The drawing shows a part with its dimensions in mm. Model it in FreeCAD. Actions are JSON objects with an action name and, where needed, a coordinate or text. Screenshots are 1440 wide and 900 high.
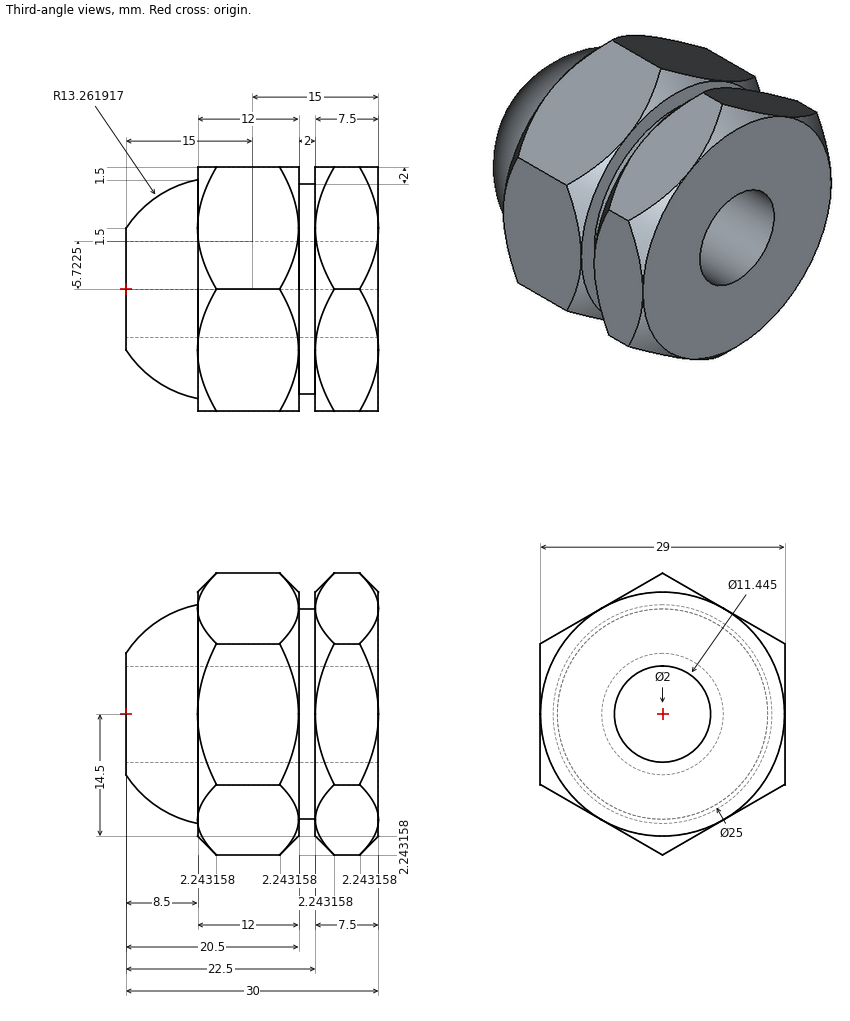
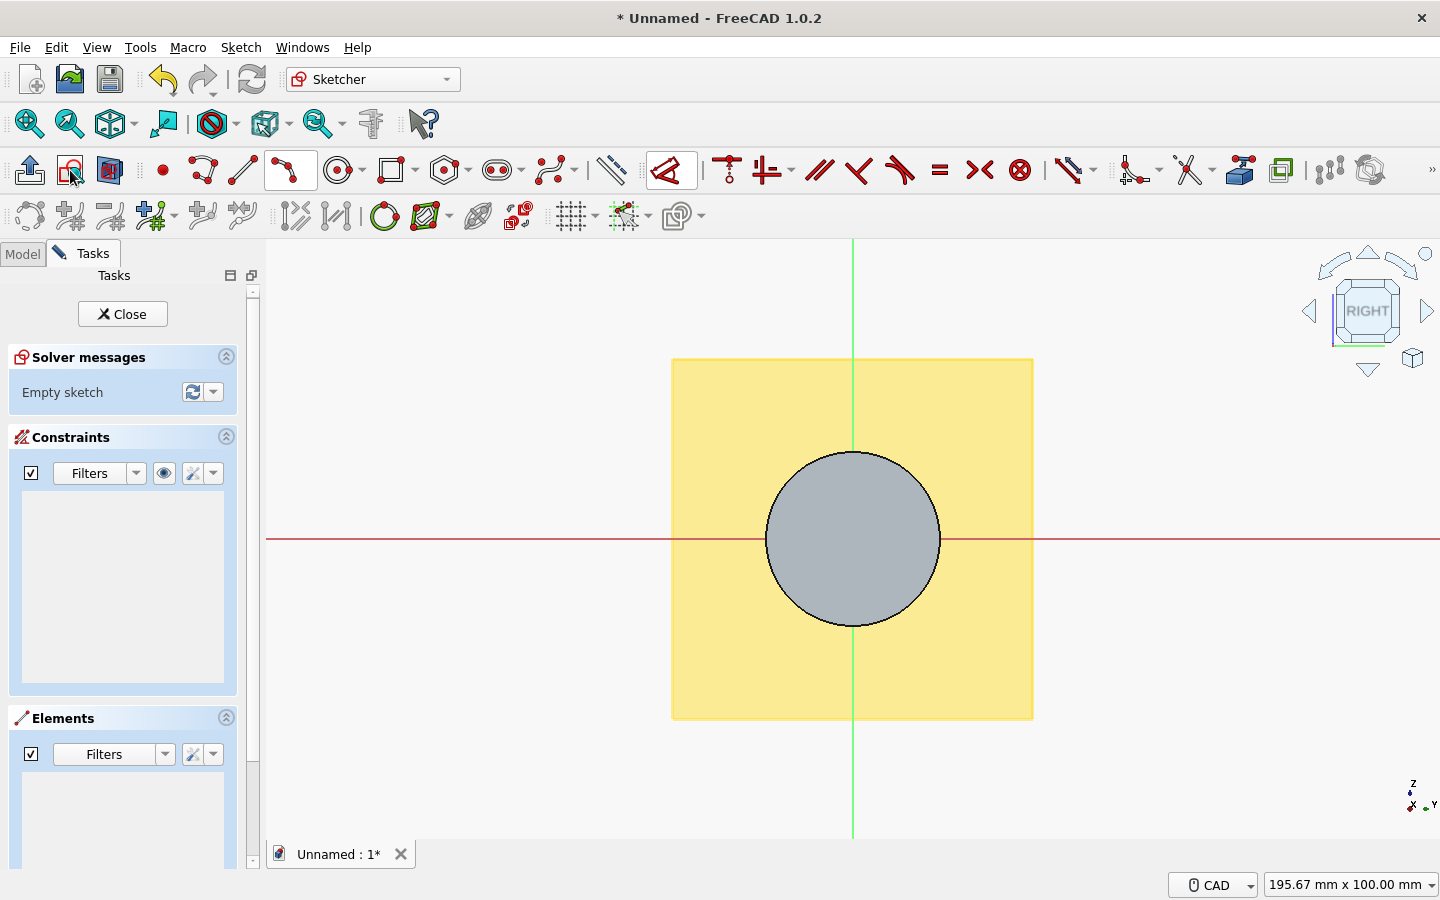
{"action": "left_click", "coordinate": [110, 170]}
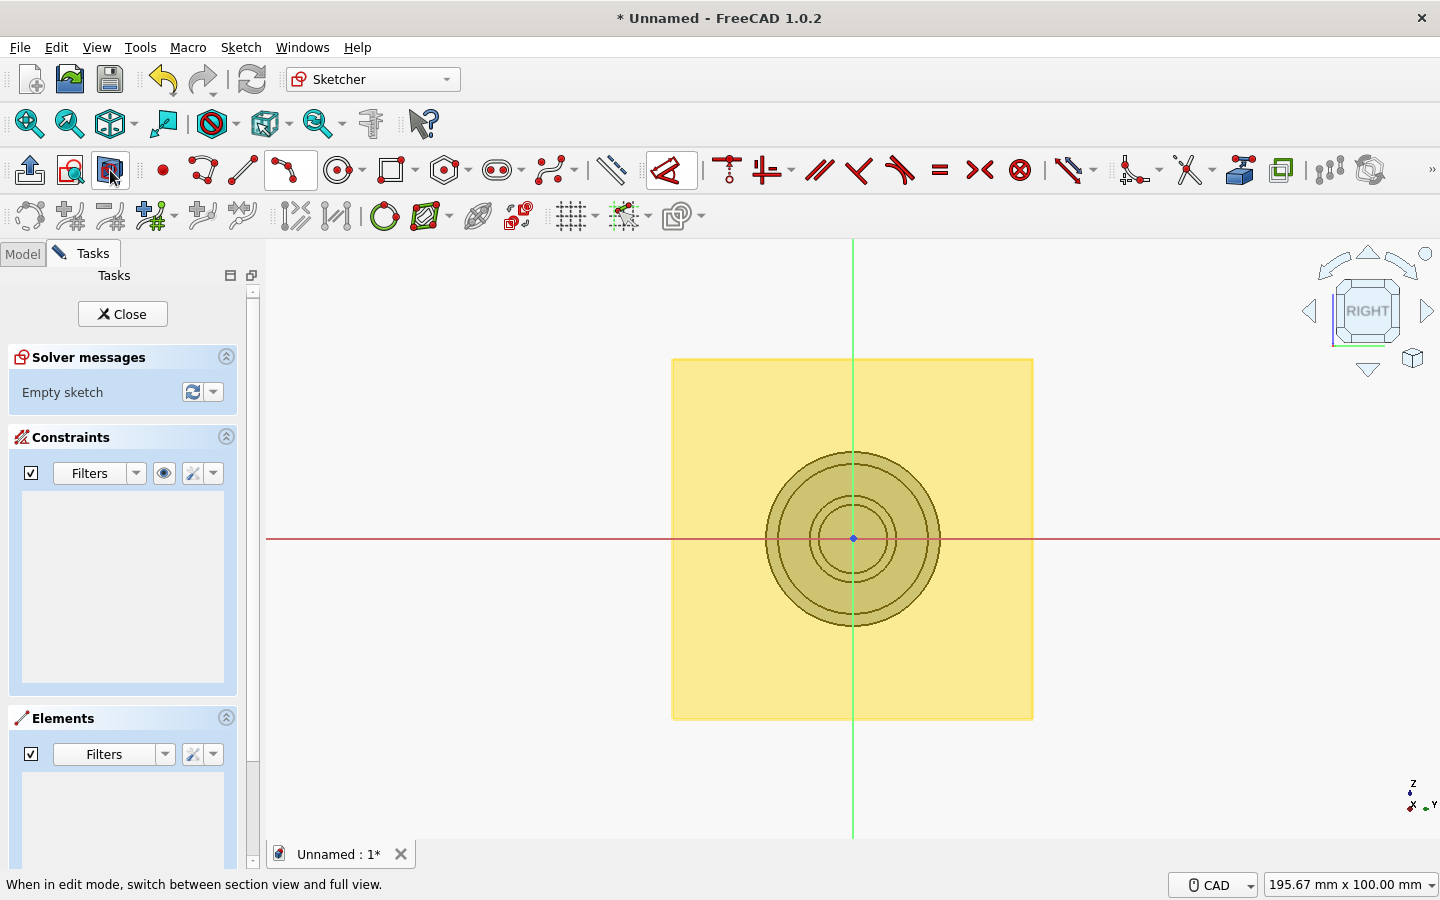
{"action": "scroll", "coordinate": [936, 539], "scroll_direction": "up", "scroll_amount": 3}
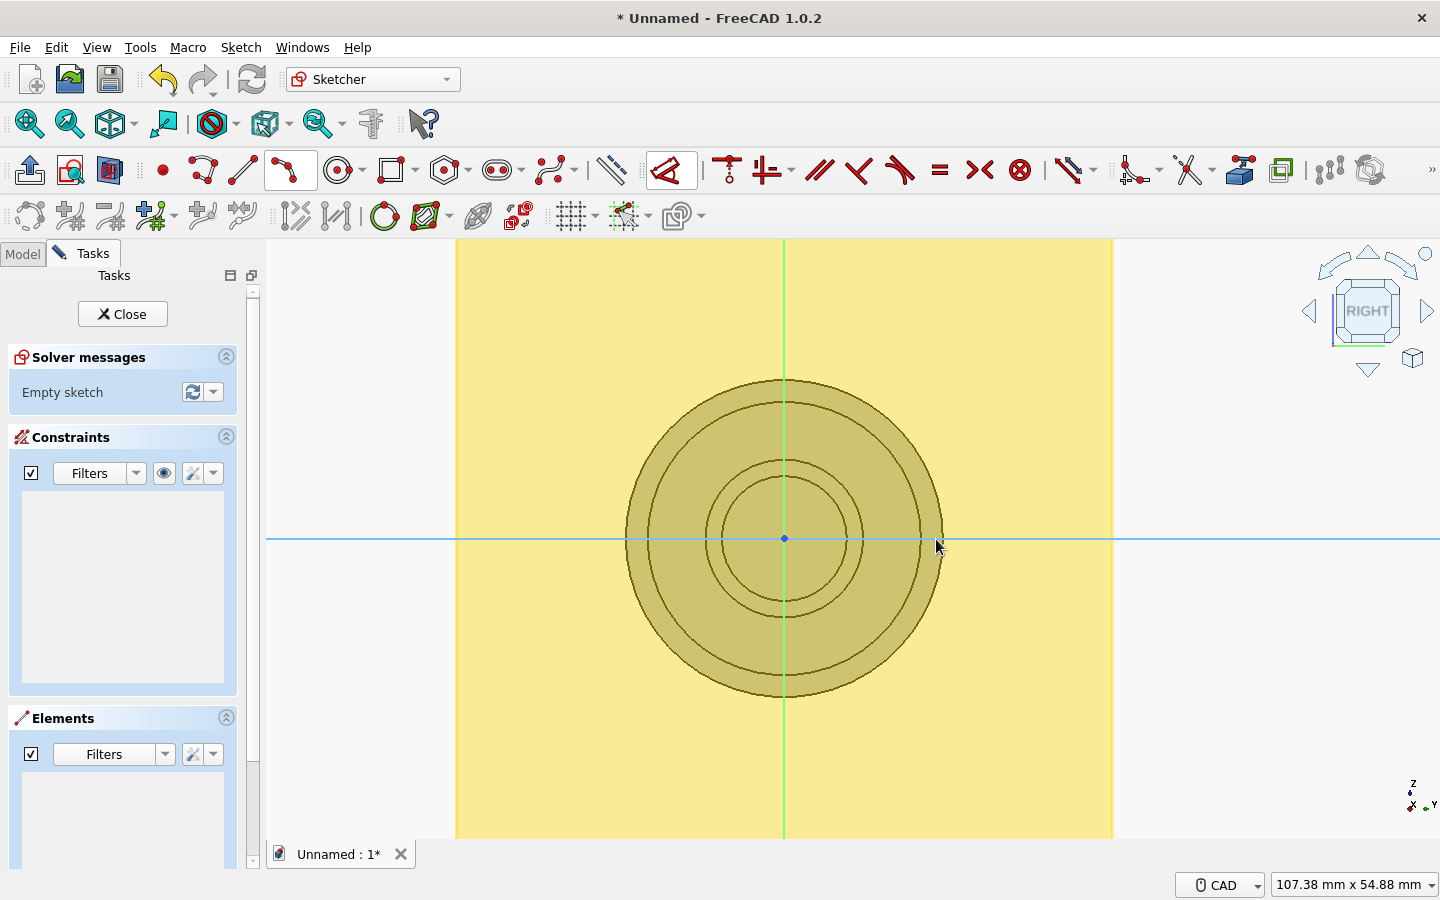
{"action": "left_click", "coordinate": [444, 170]}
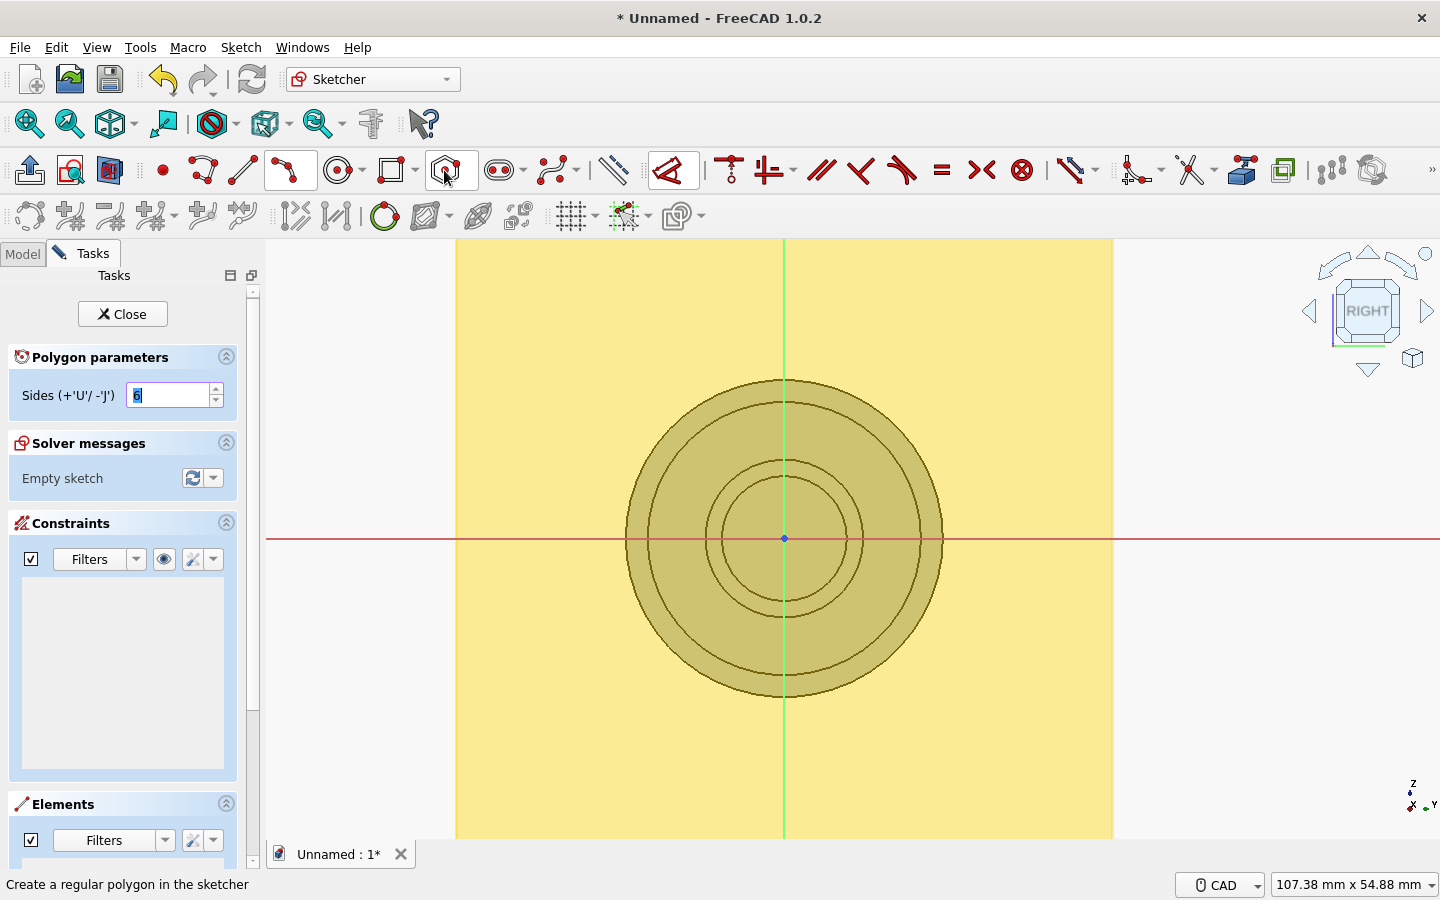
{"action": "left_click", "coordinate": [784, 539]}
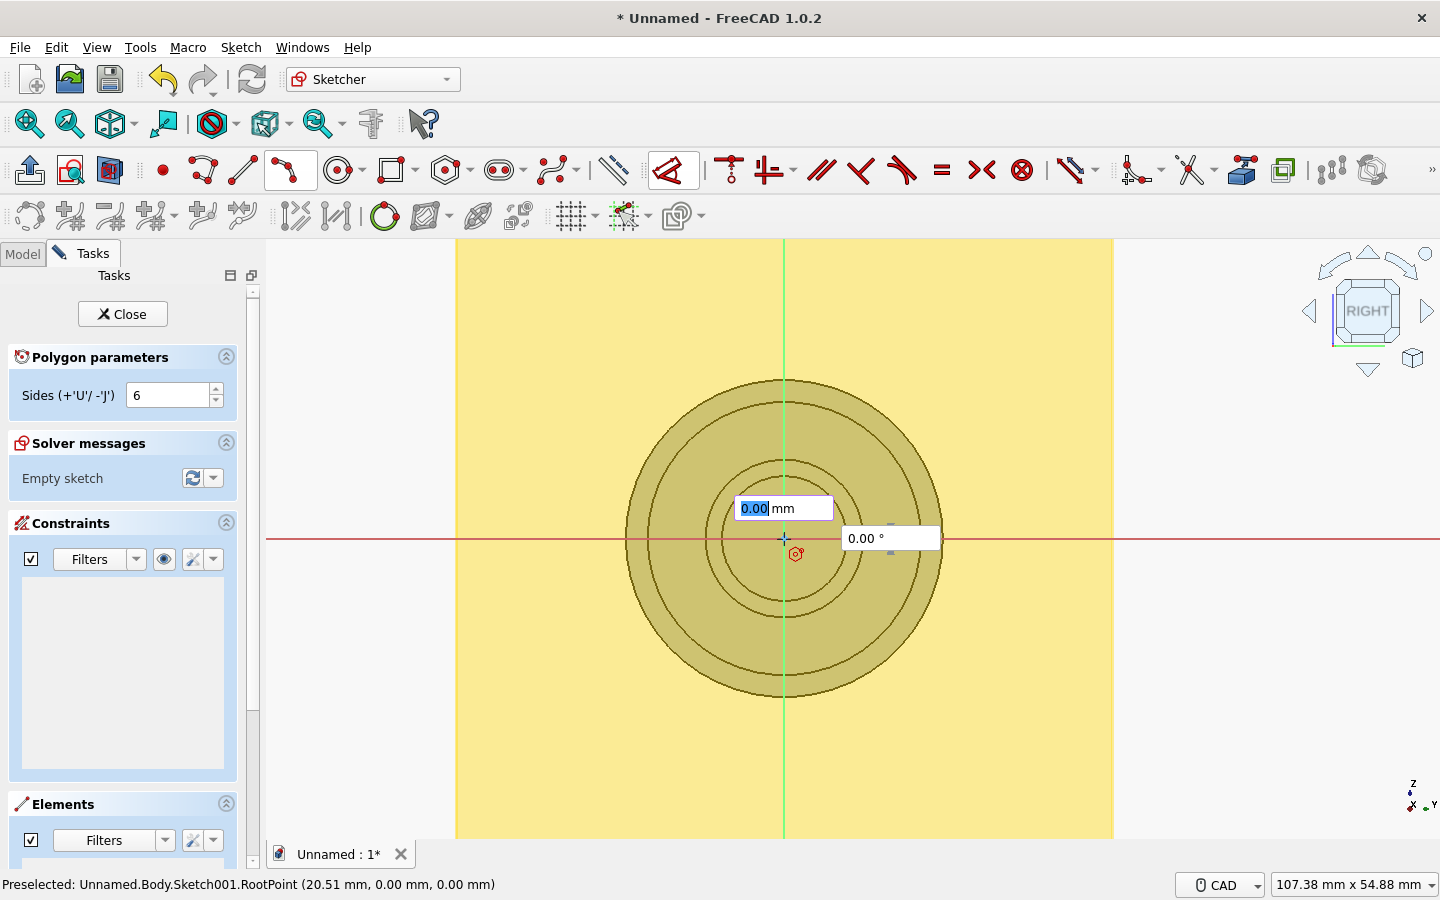
{"action": "left_click", "coordinate": [784, 722]}
{"action": "key", "text": "Escape"}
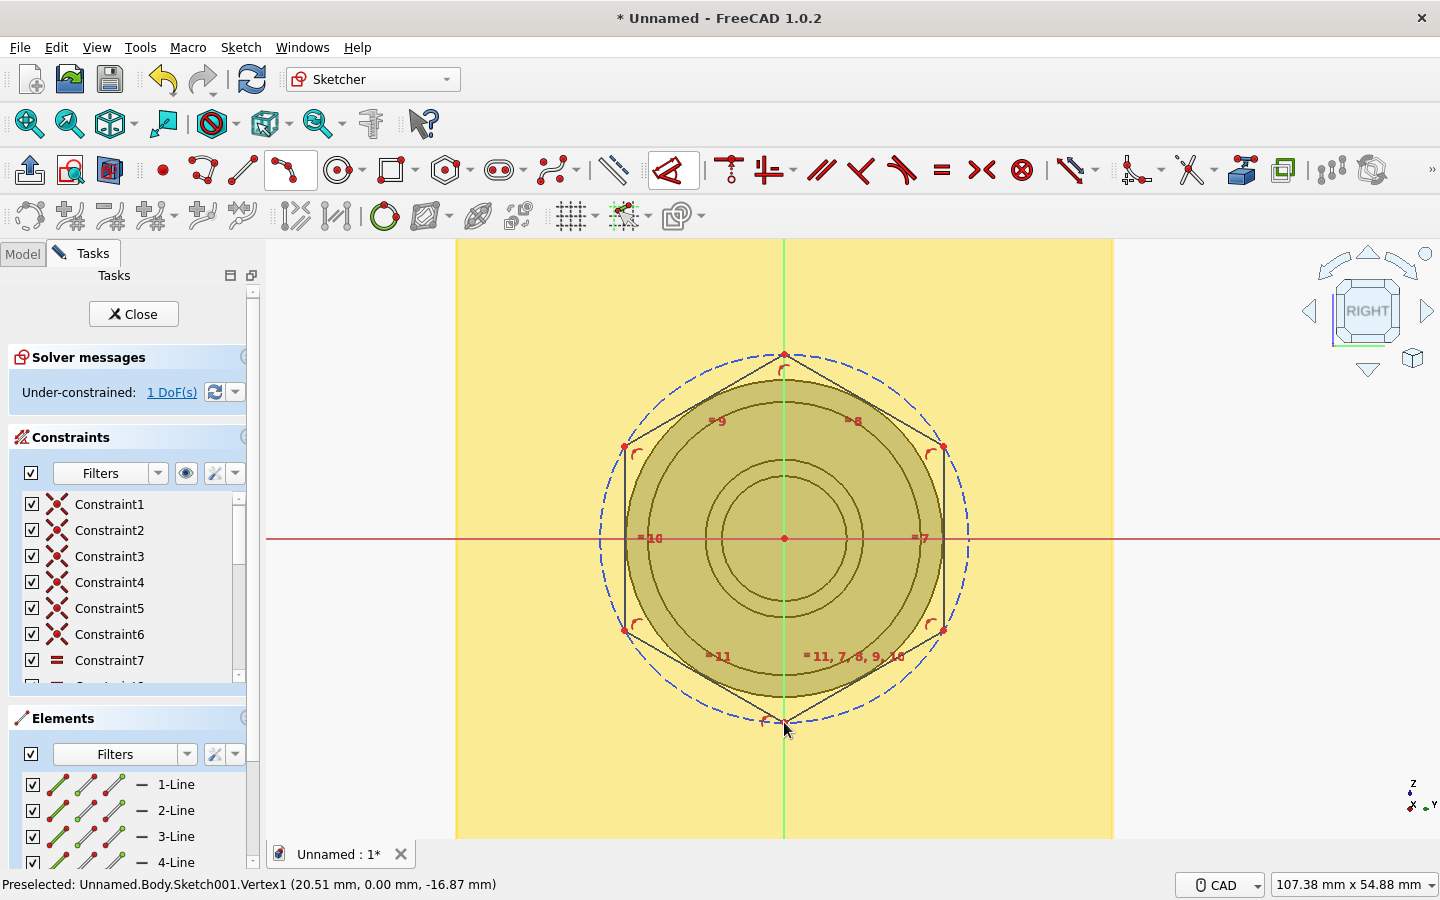
{"action": "key", "text": "g c"}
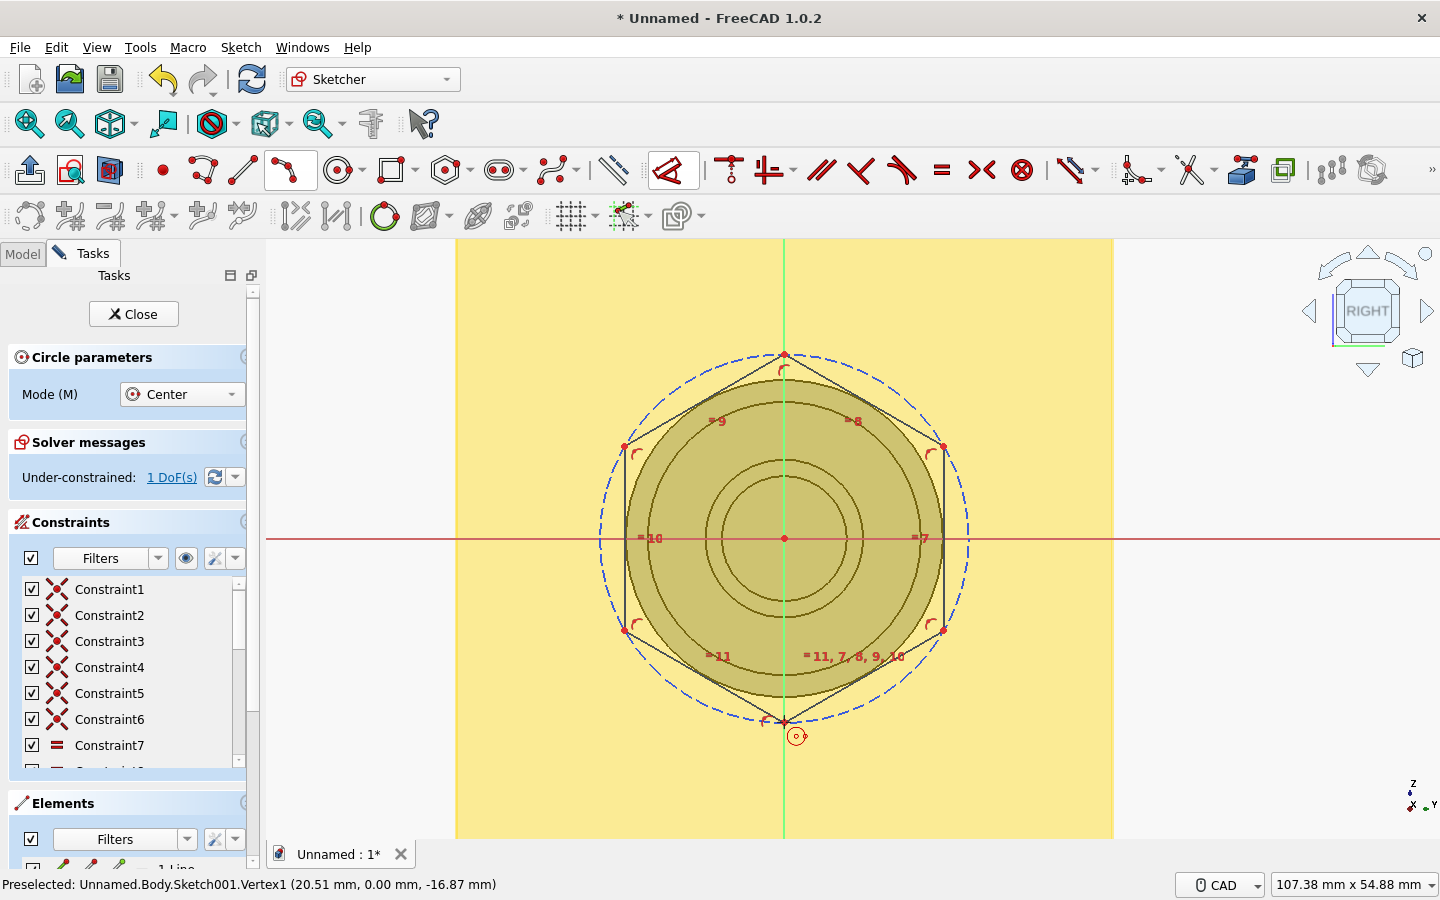
{"action": "left_click", "coordinate": [784, 539]}
{"action": "left_click", "coordinate": [881, 442]}
{"action": "key", "text": "Escape"}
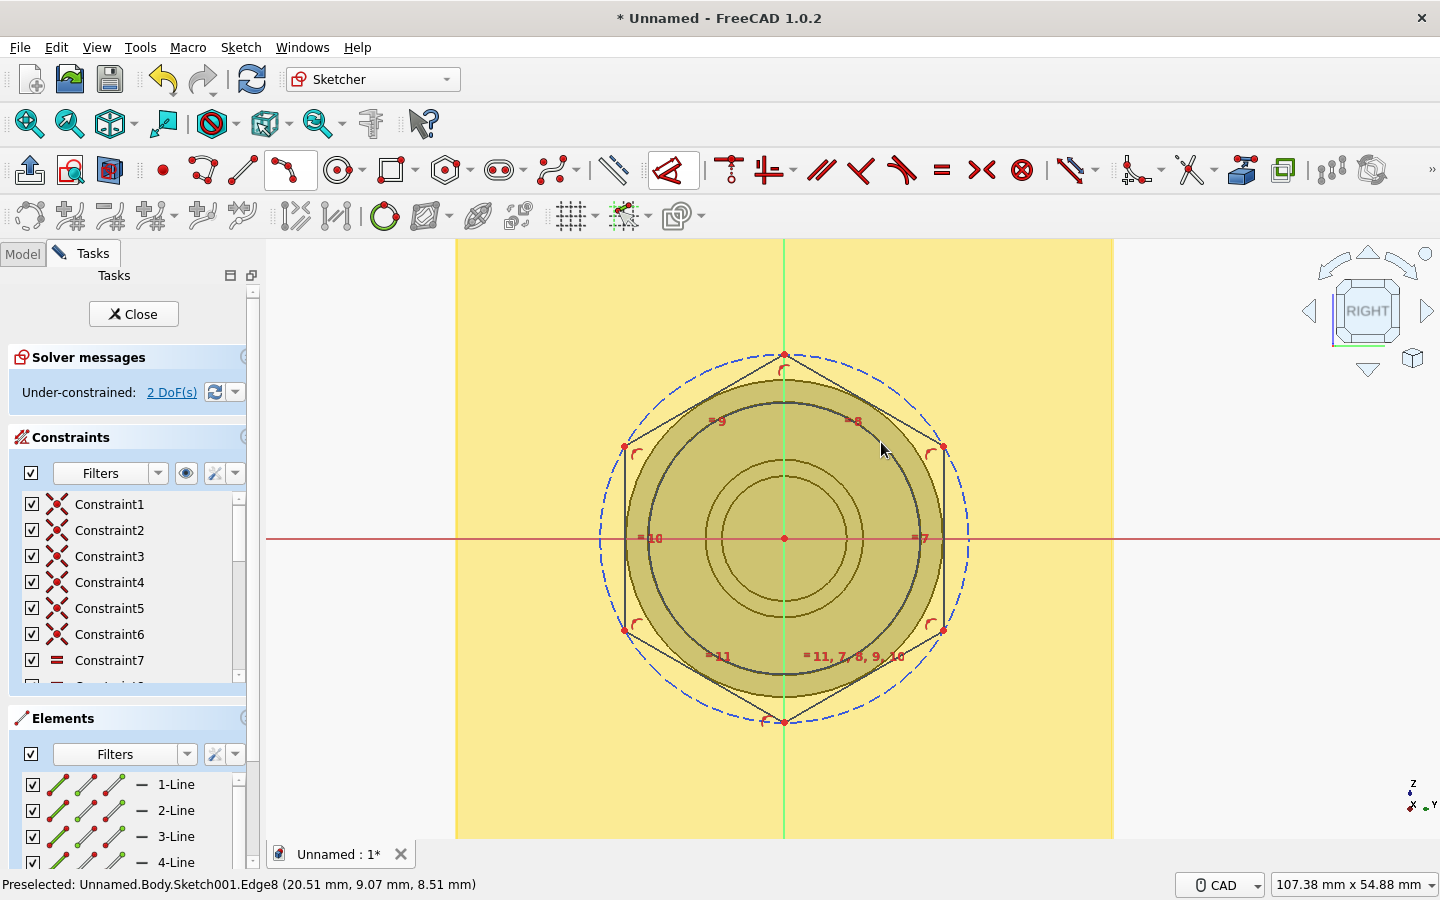
{"action": "left_click", "coordinate": [880, 442]}